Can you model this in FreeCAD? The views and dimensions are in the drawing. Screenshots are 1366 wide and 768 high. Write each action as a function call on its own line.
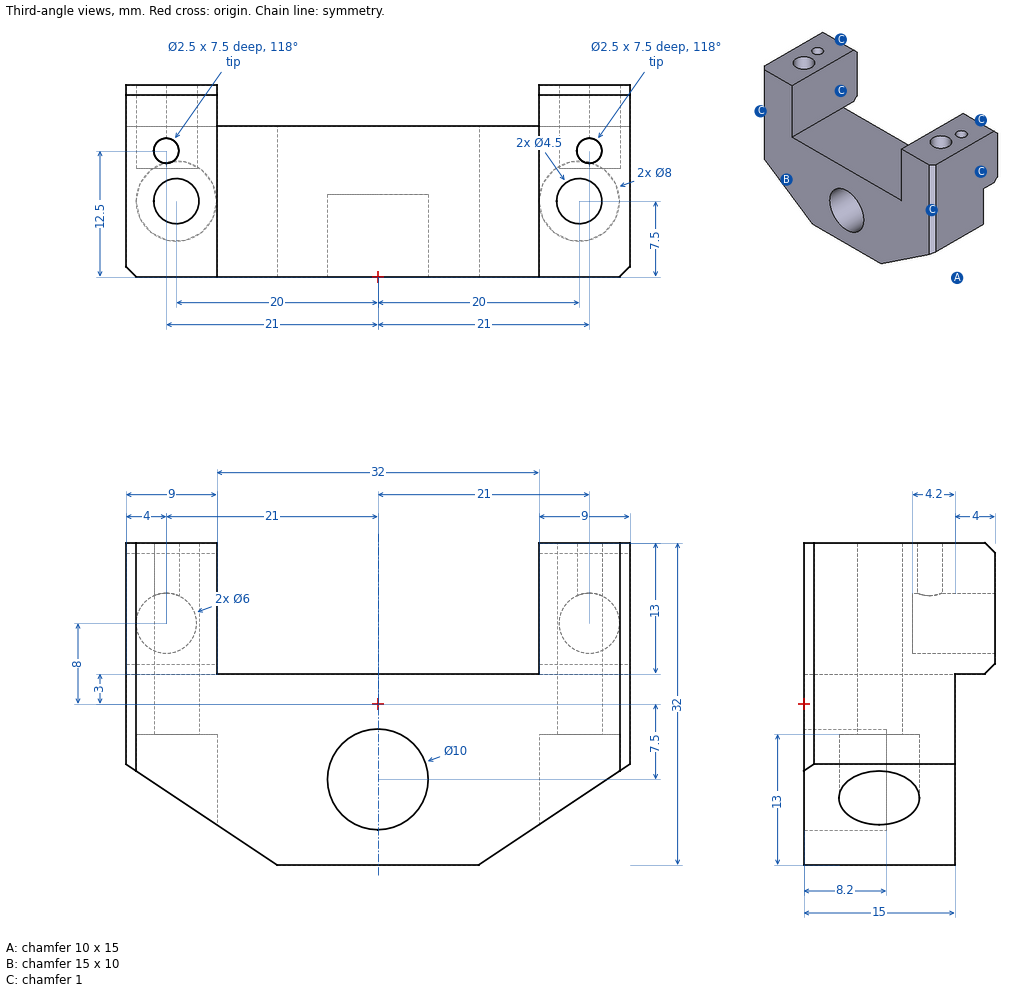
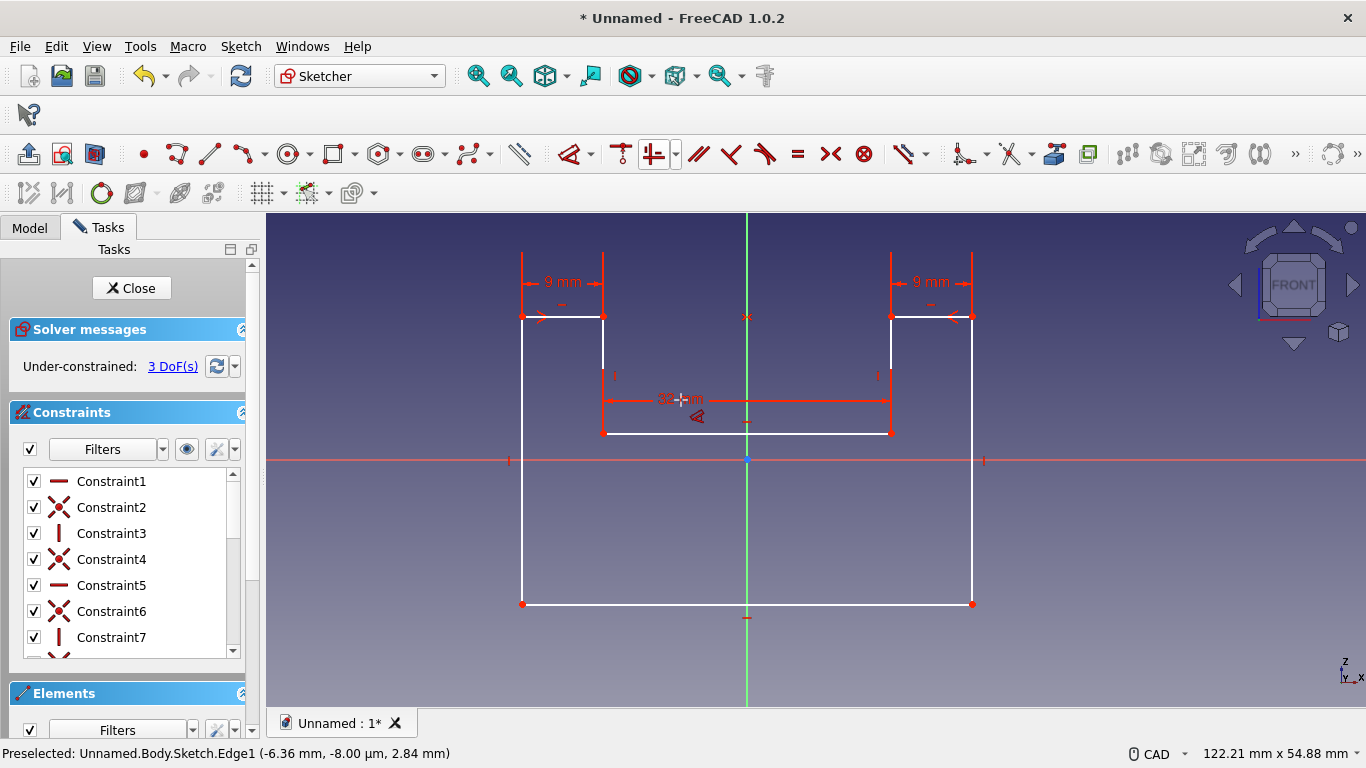
click(891, 399)
click(925, 375)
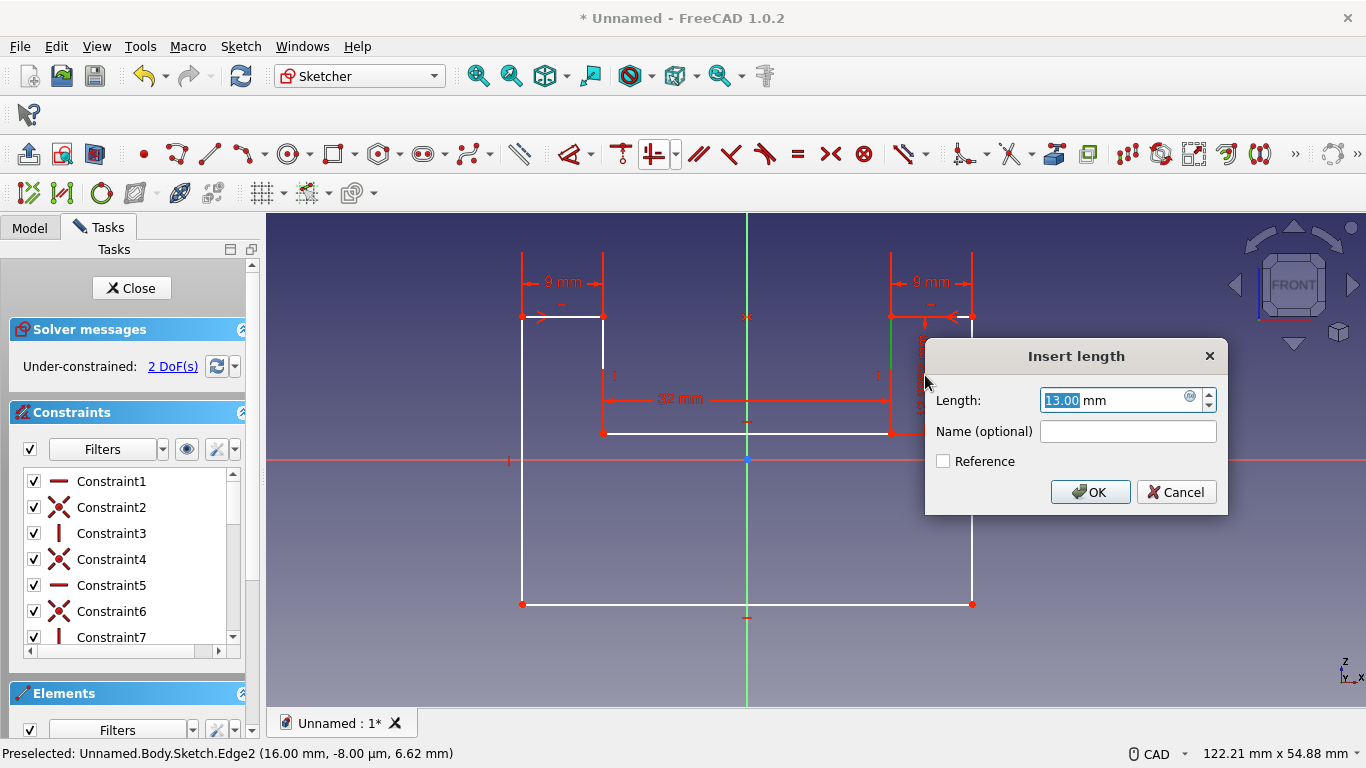
text(13)
key(Return)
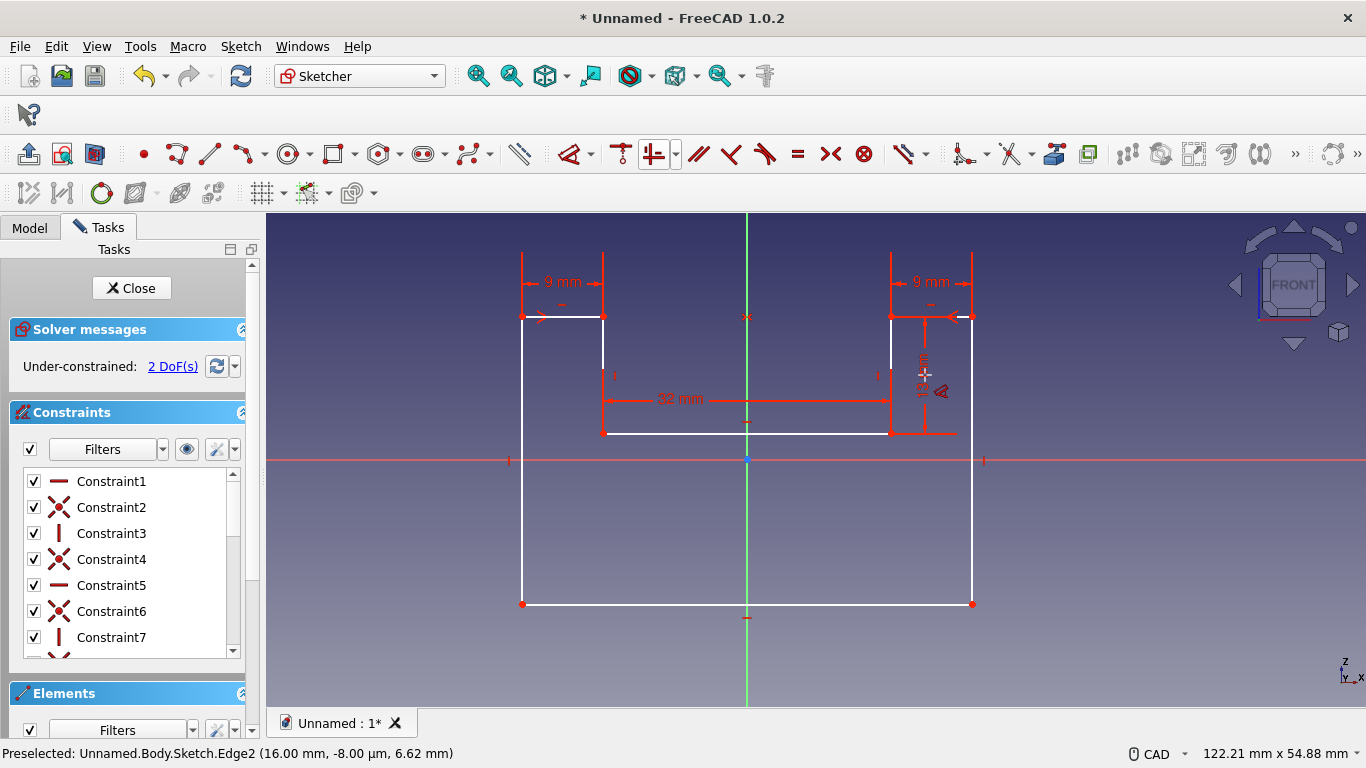
click(972, 403)
click(1006, 395)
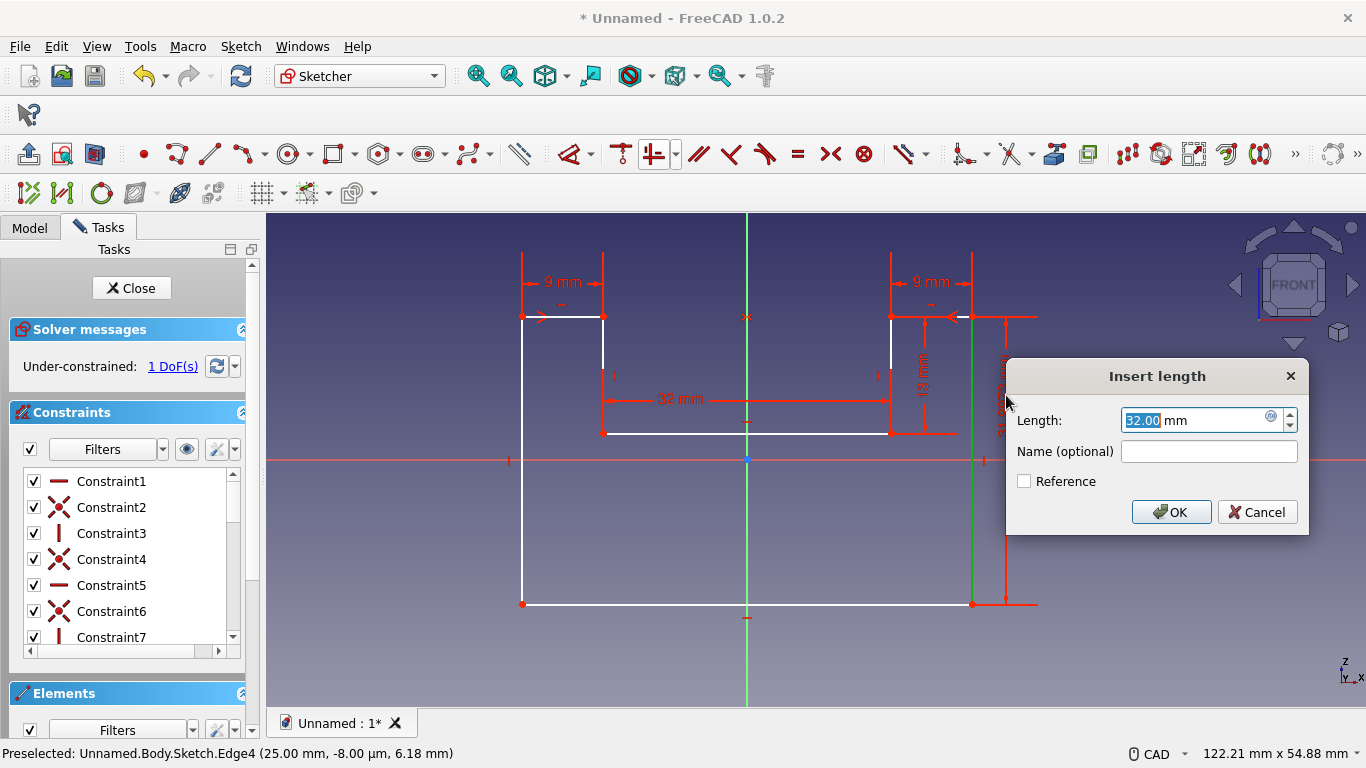
text(32)
key(Return)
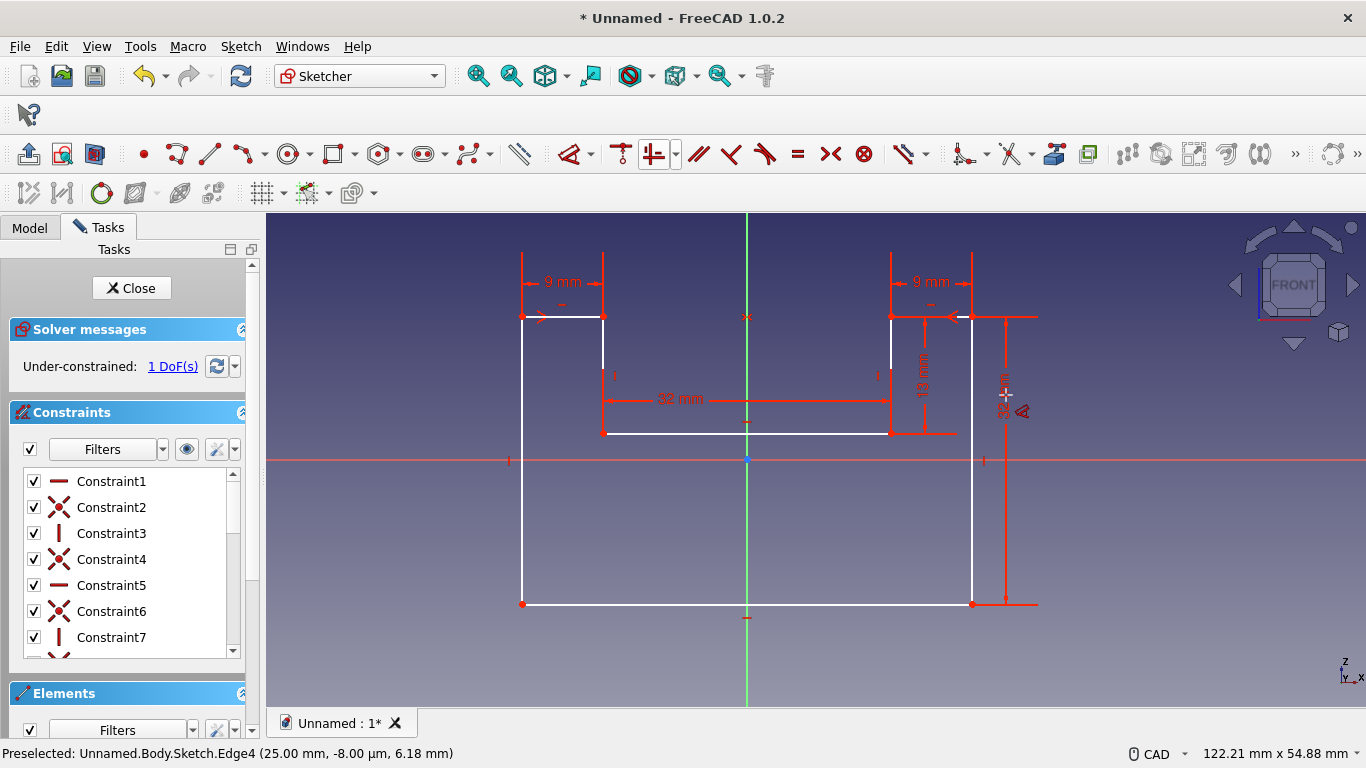
scroll(603, 434, up, 2)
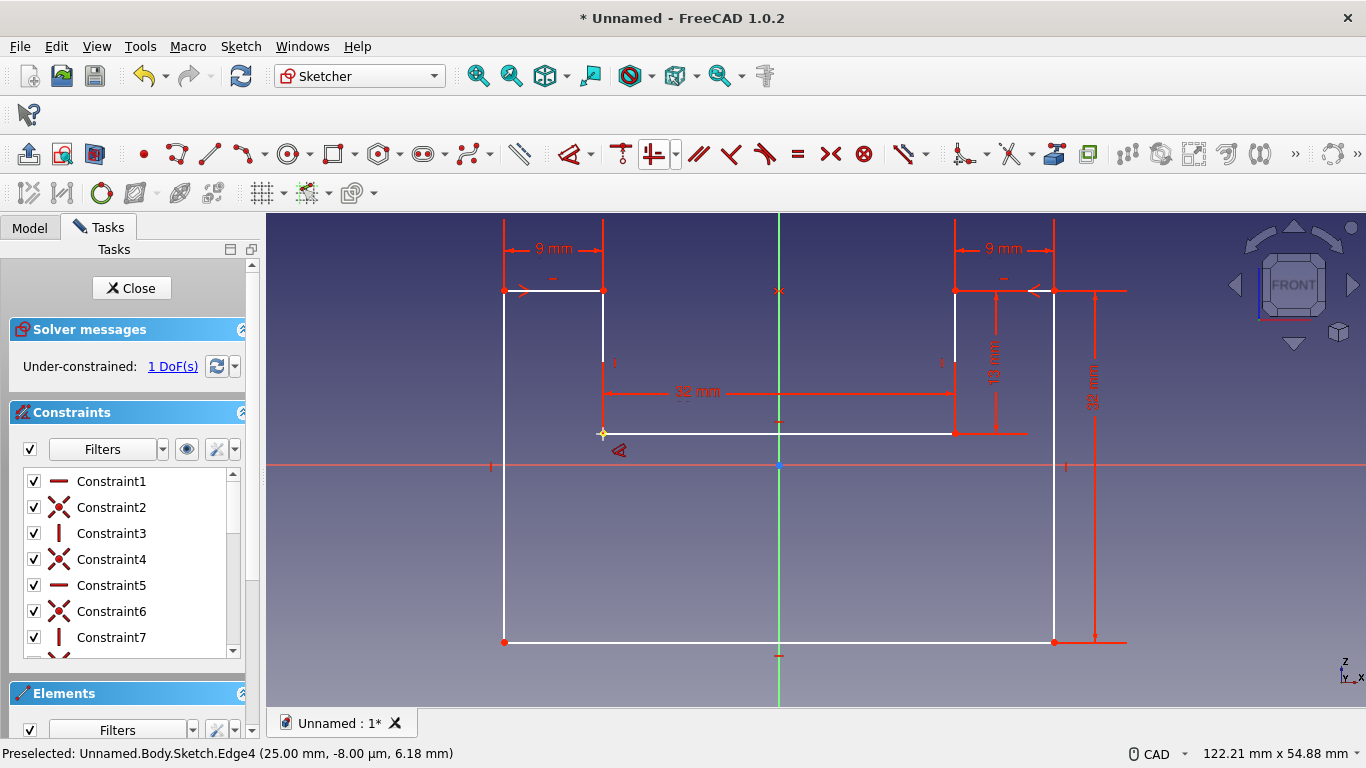
click(603, 434)
click(569, 453)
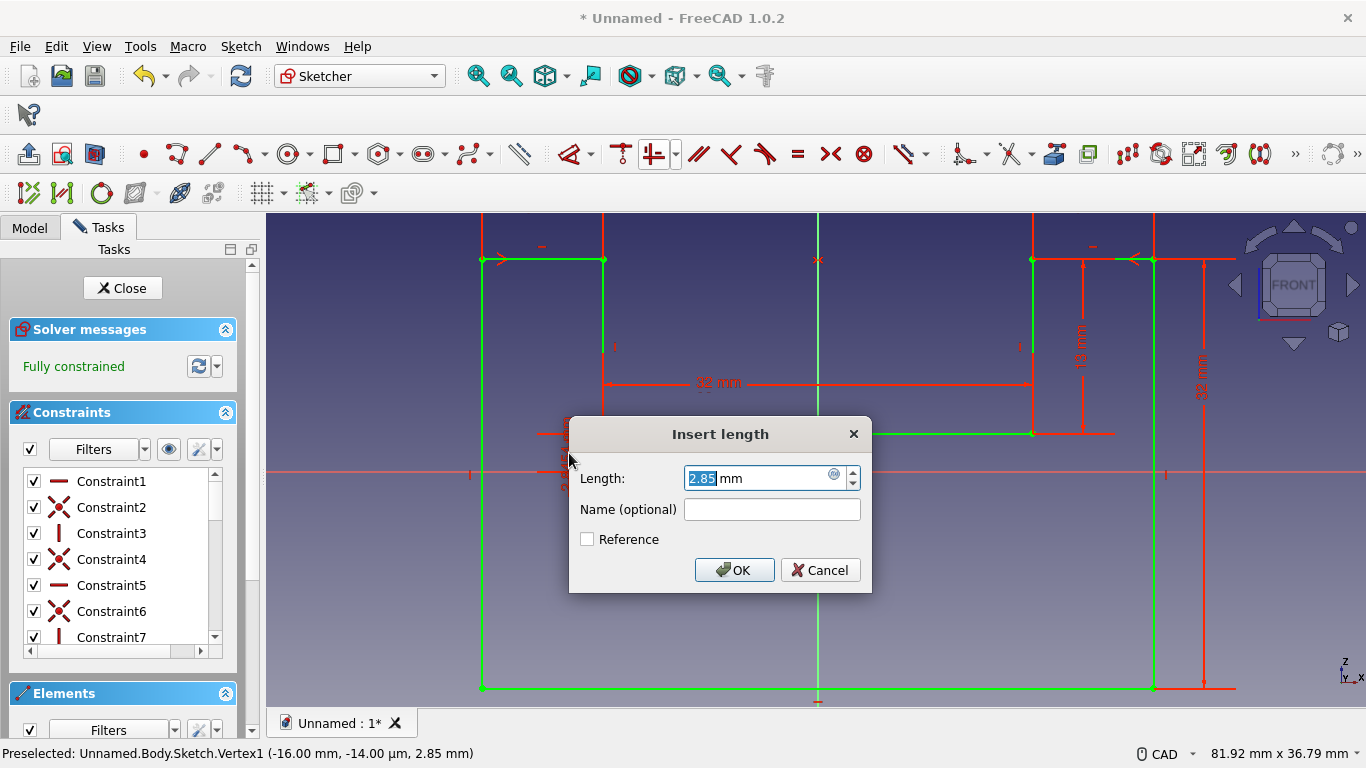
text(3)
key(Return)
key(Escape)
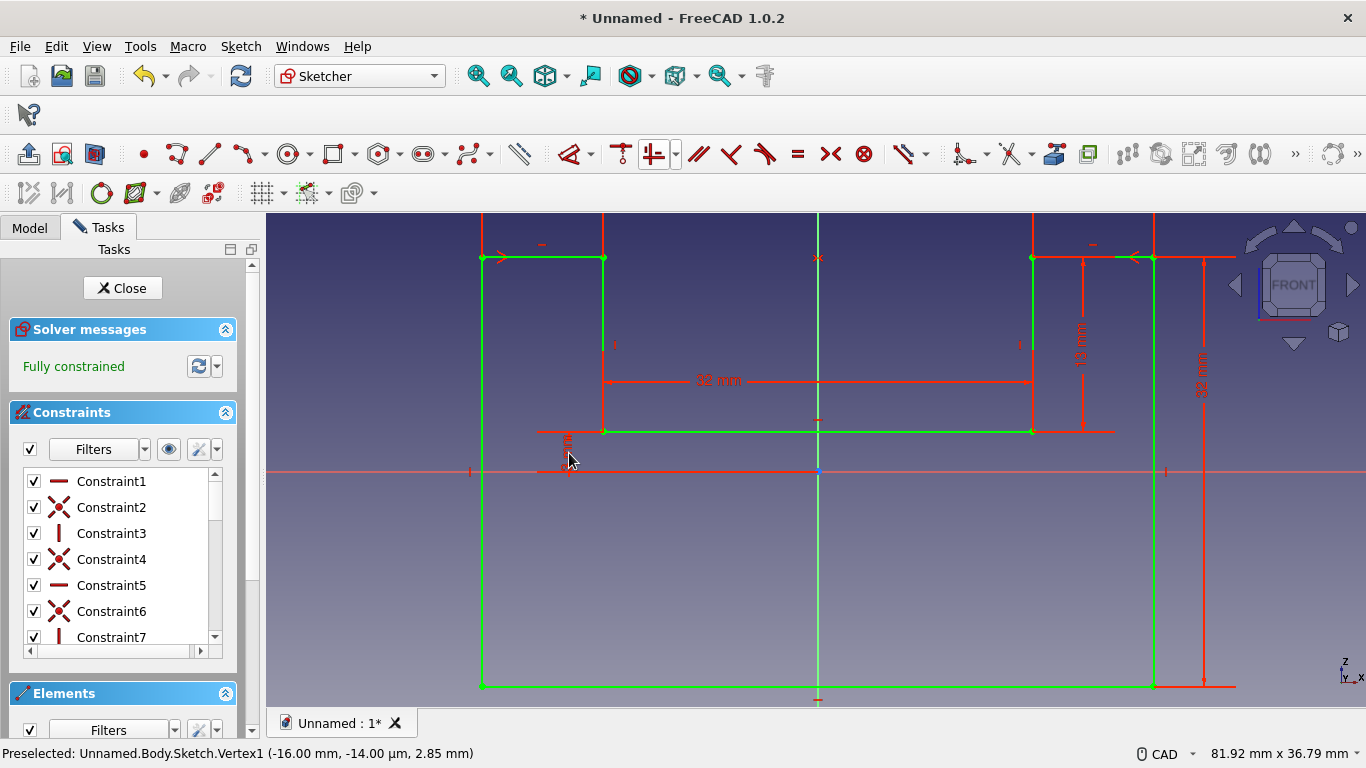
click(123, 288)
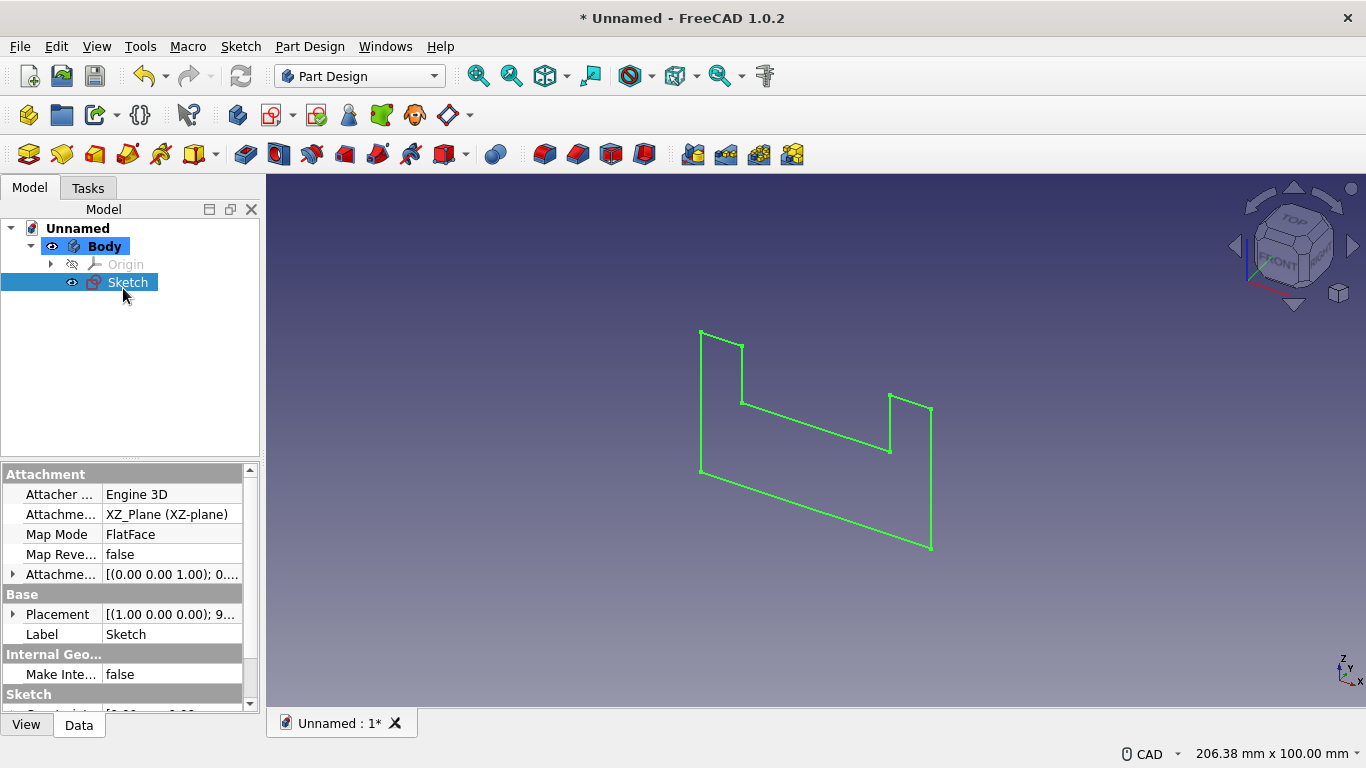
click(29, 154)